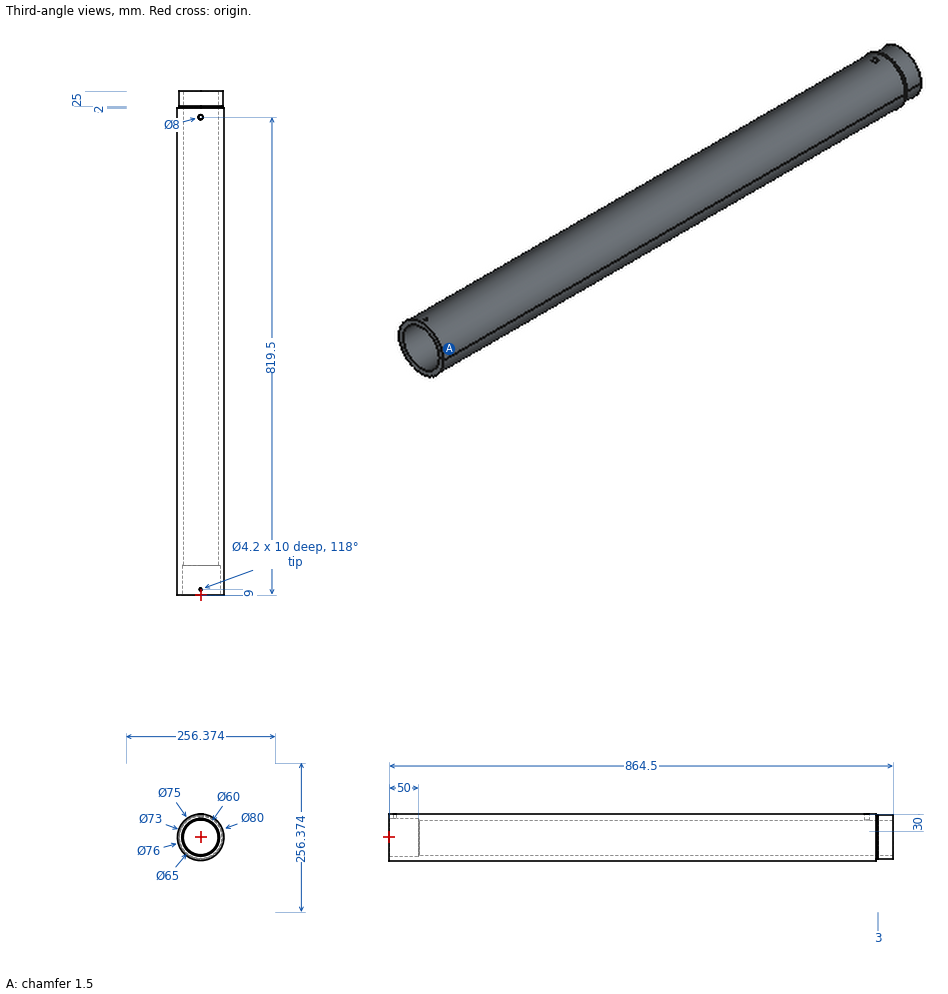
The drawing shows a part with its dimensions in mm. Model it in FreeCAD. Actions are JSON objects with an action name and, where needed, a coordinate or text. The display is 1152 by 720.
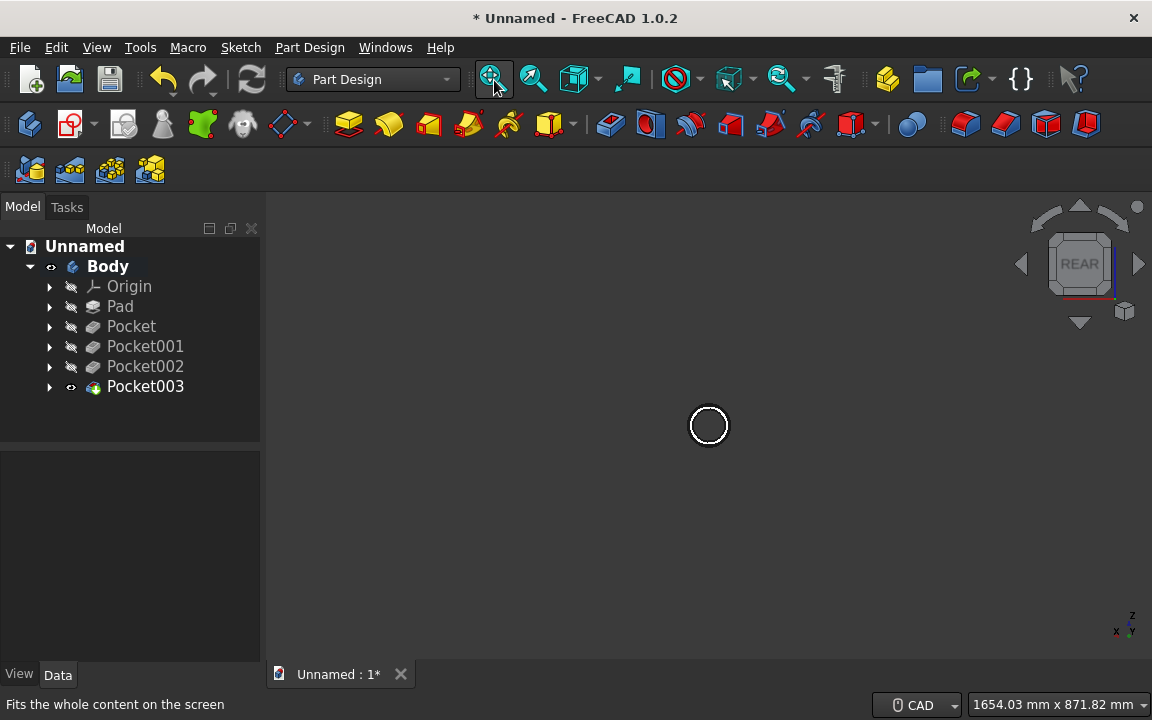
{"action": "left_click", "coordinate": [494, 80]}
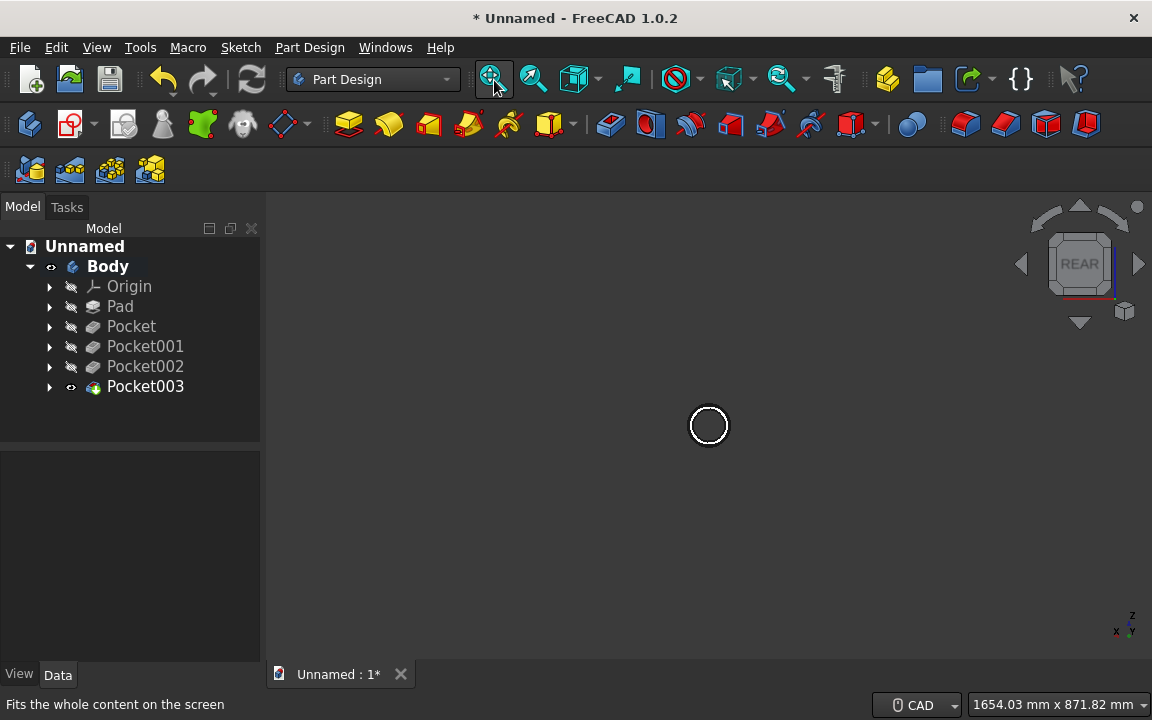
{"action": "key", "text": "6"}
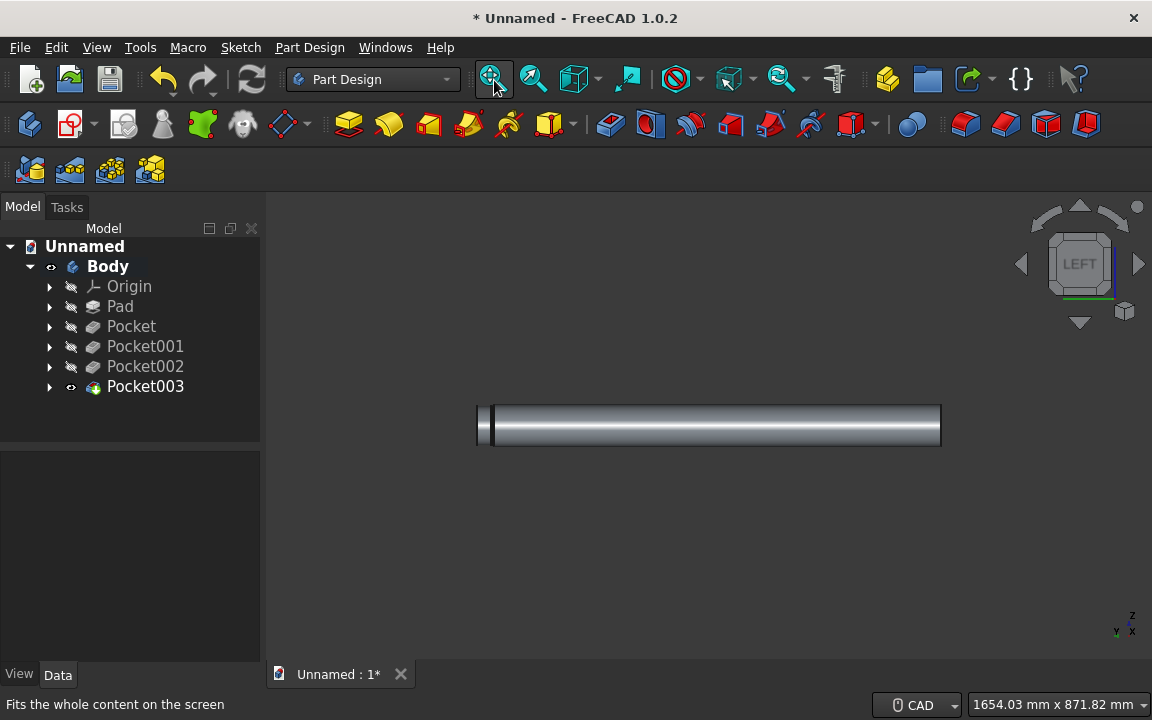
{"action": "key", "text": "v 3"}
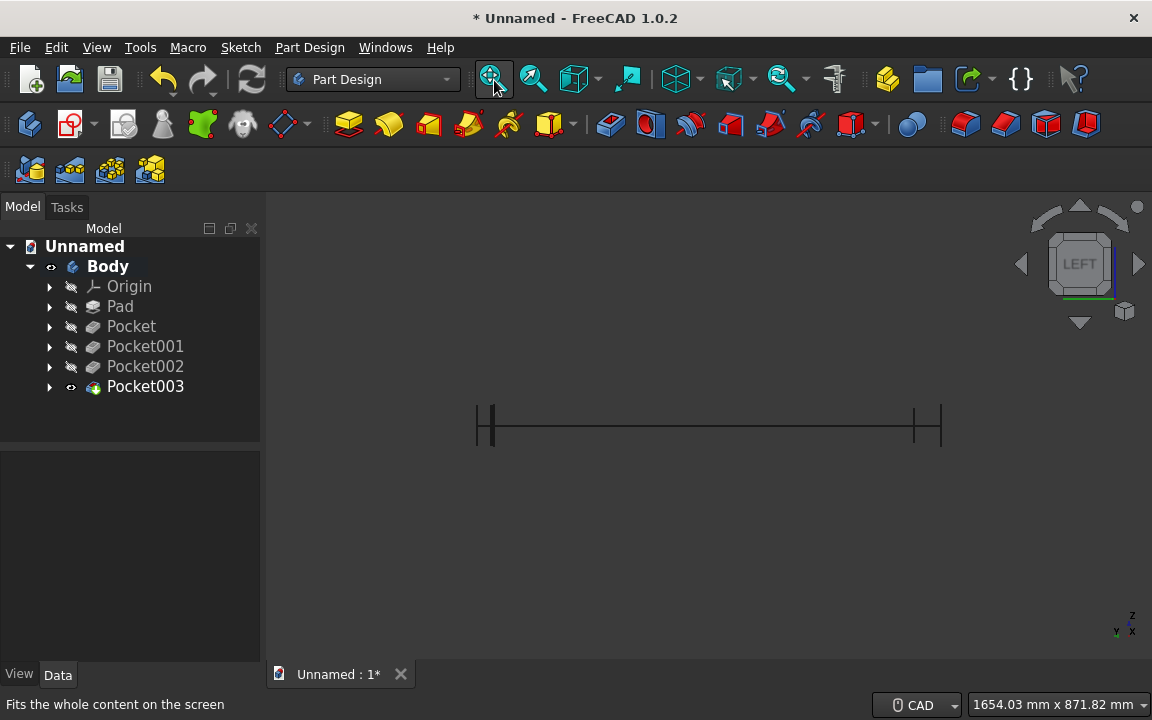
{"action": "key", "text": "0"}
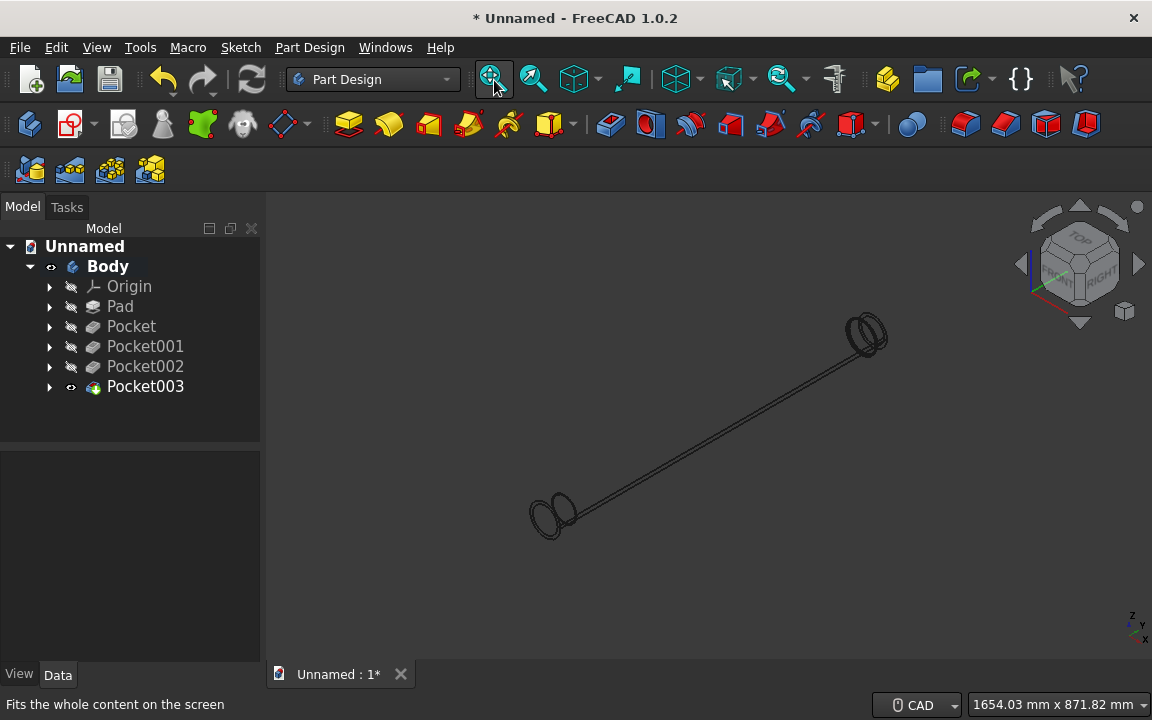
{"action": "scroll", "coordinate": [553, 502], "scroll_direction": "up", "scroll_amount": 6}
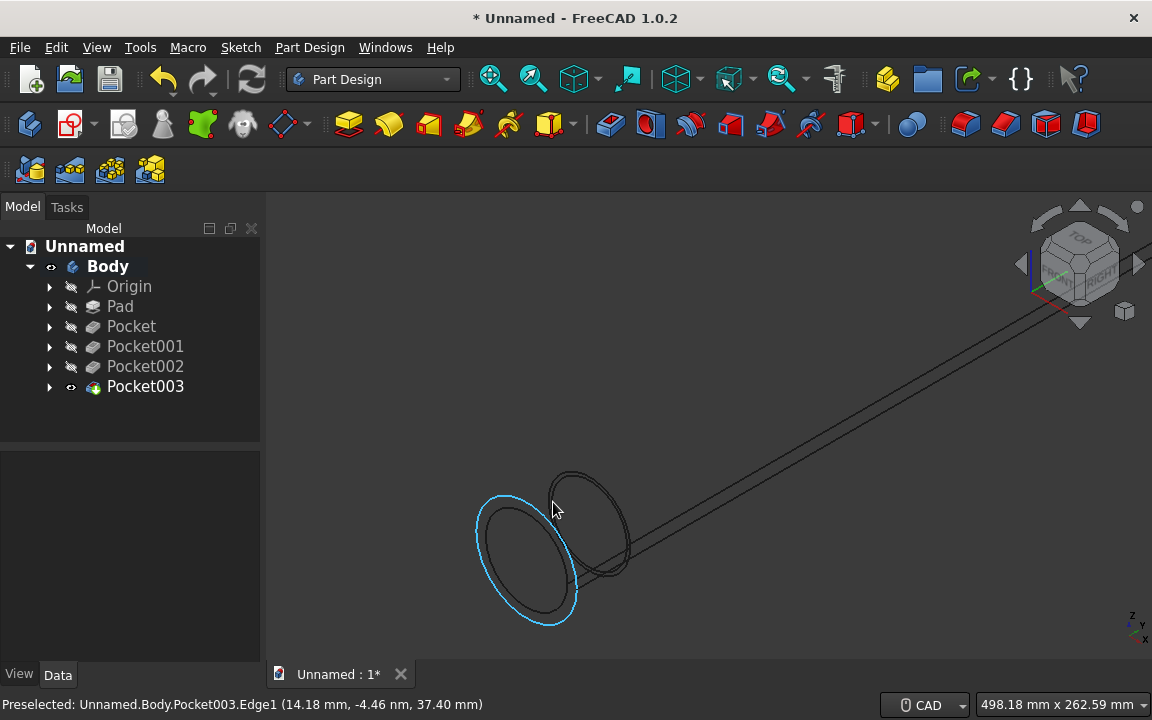
{"action": "left_click", "coordinate": [552, 501]}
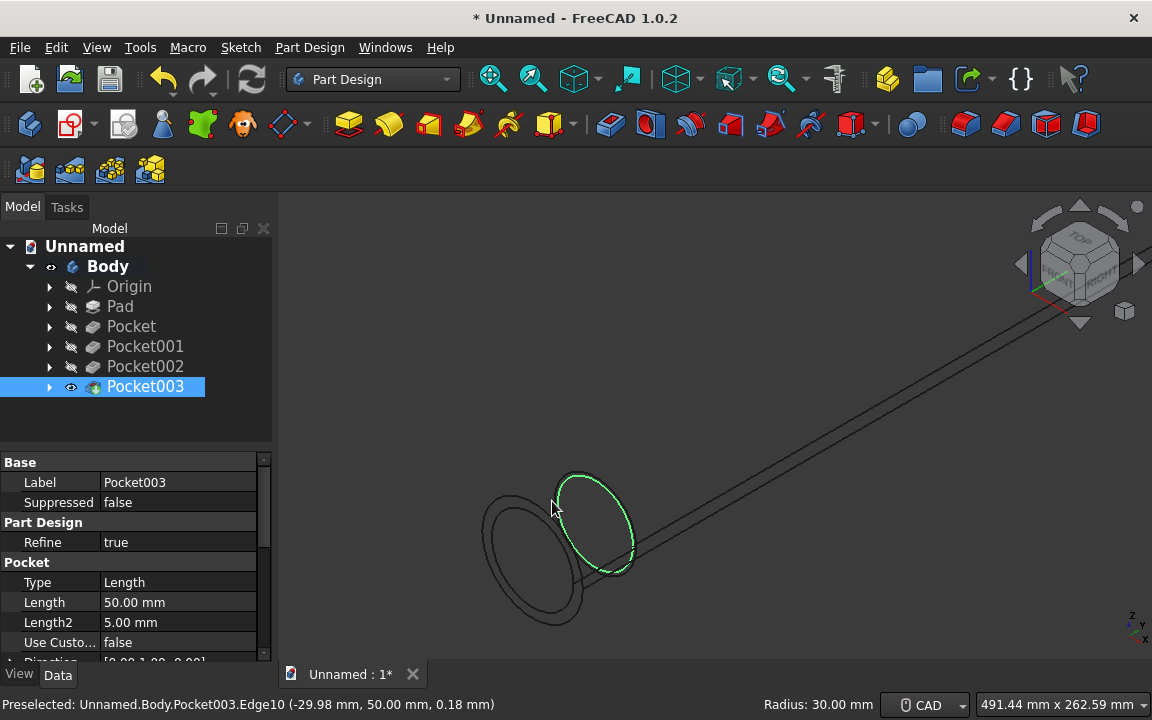
{"action": "key", "text": "v 1"}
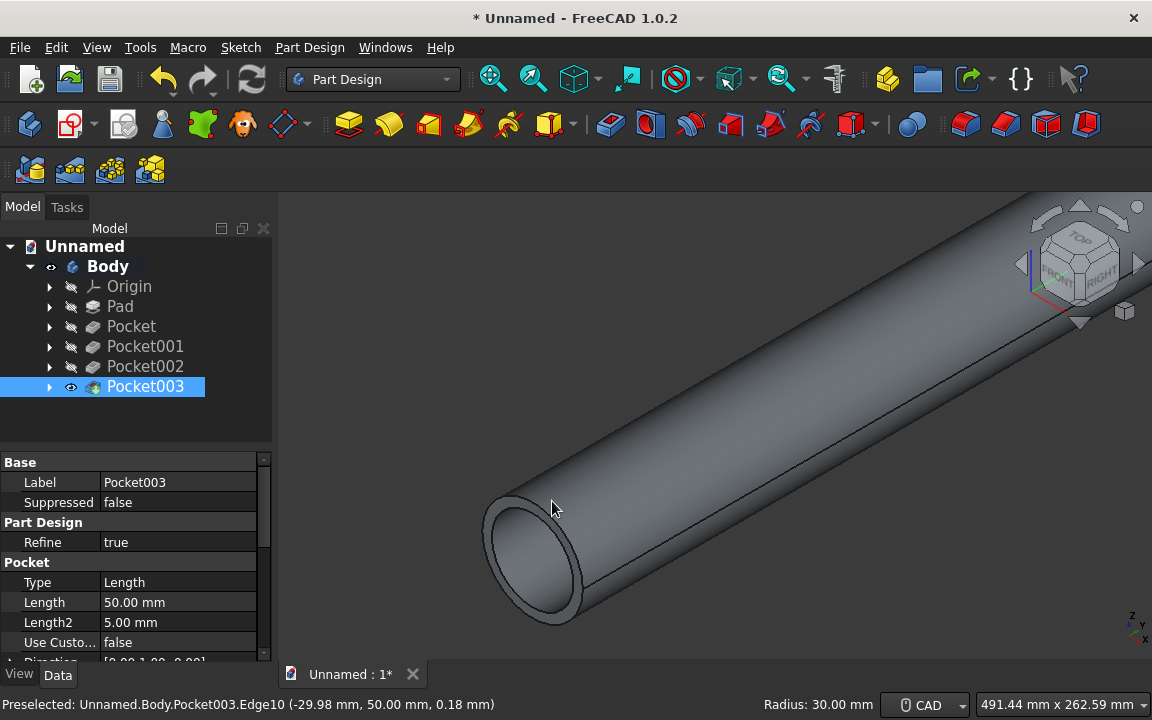
{"action": "left_click", "coordinate": [1006, 124]}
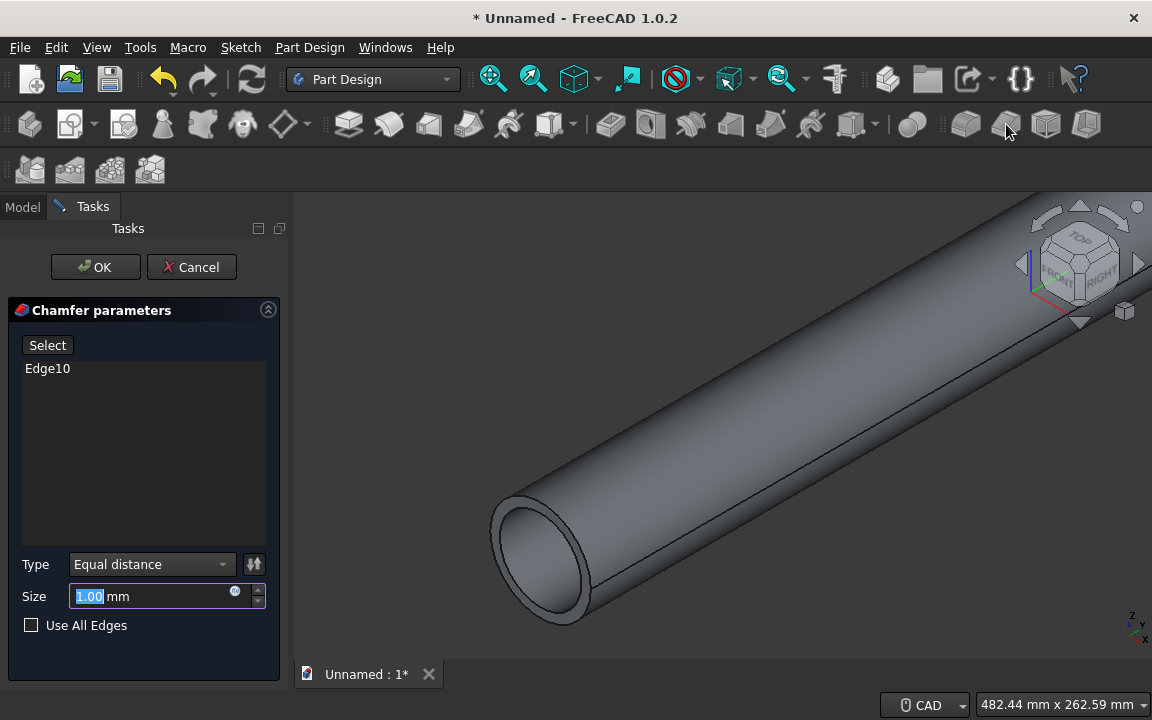
{"action": "type", "text": "1.5"}
{"action": "key", "text": "Tab"}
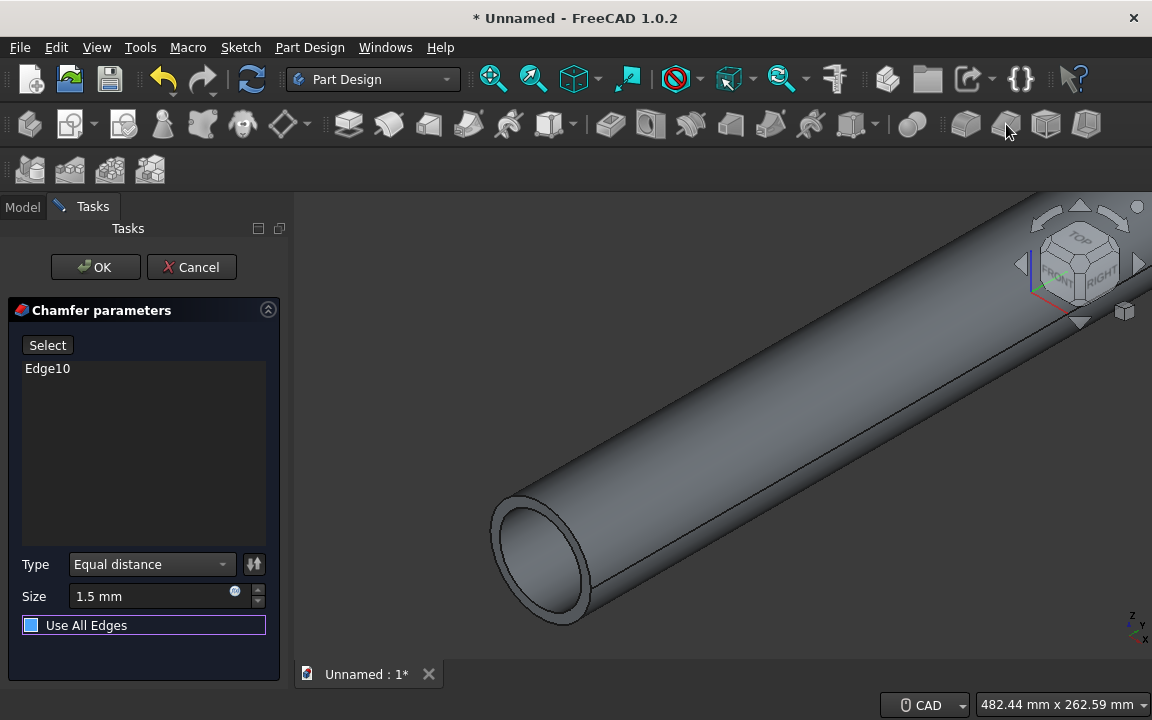
{"action": "left_click", "coordinate": [96, 267]}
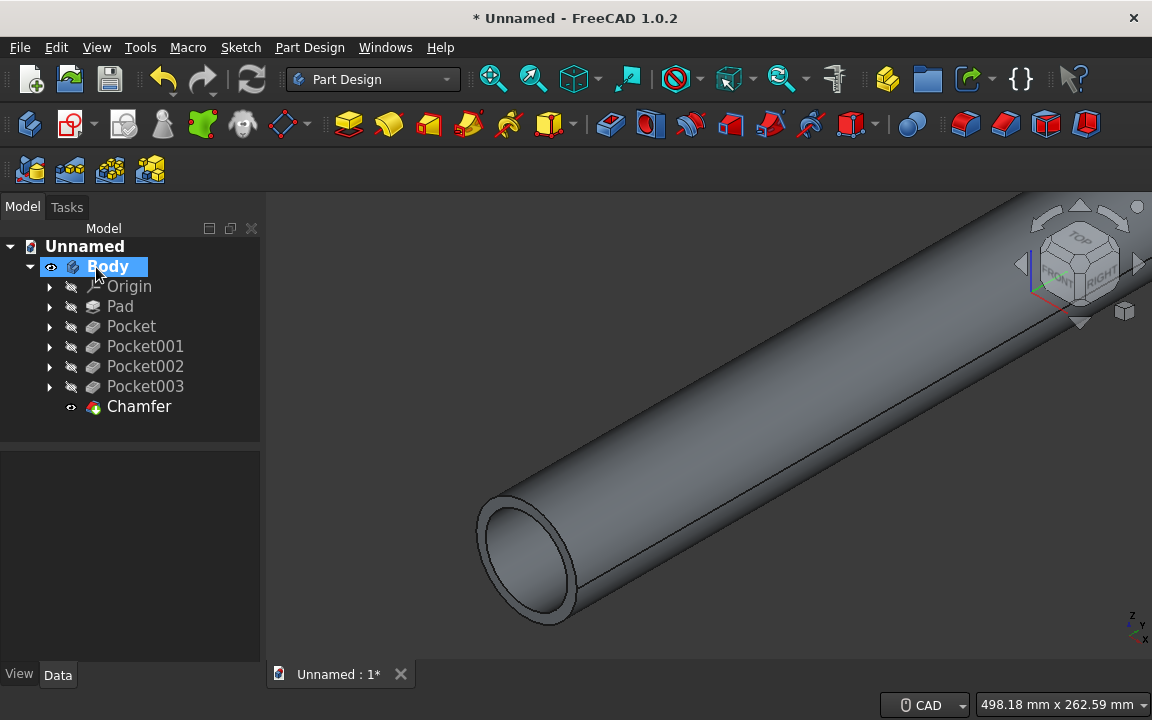
{"action": "key", "text": "v f"}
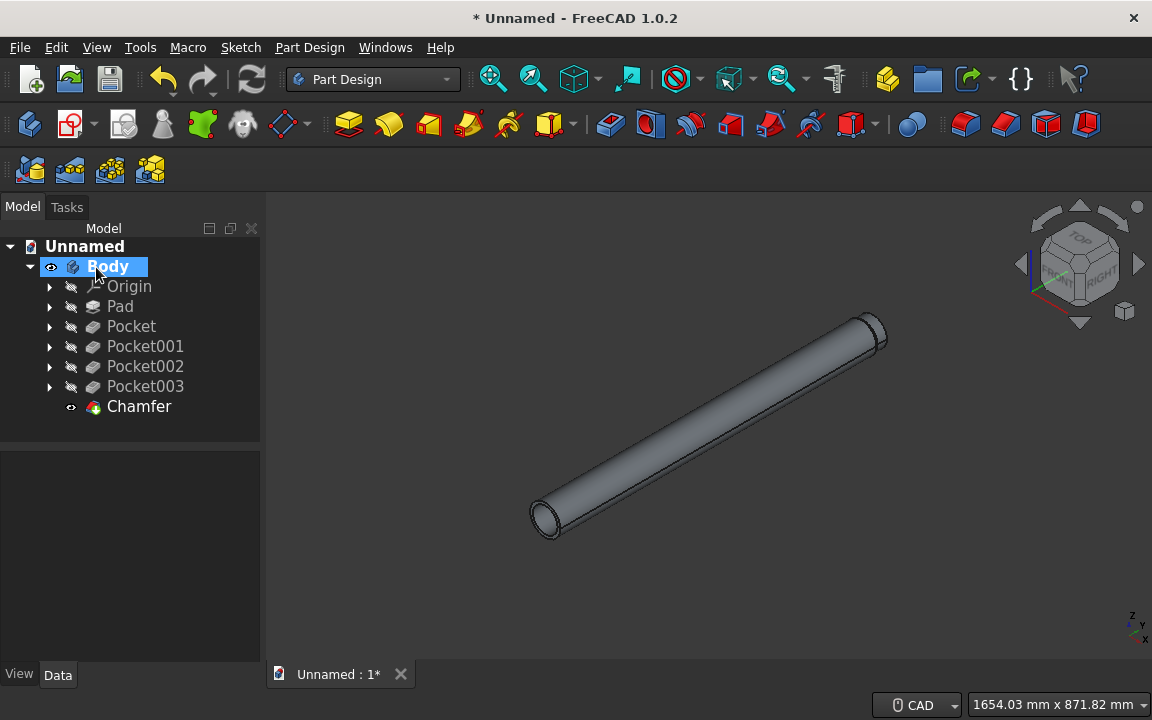
{"action": "left_click", "coordinate": [50, 287]}